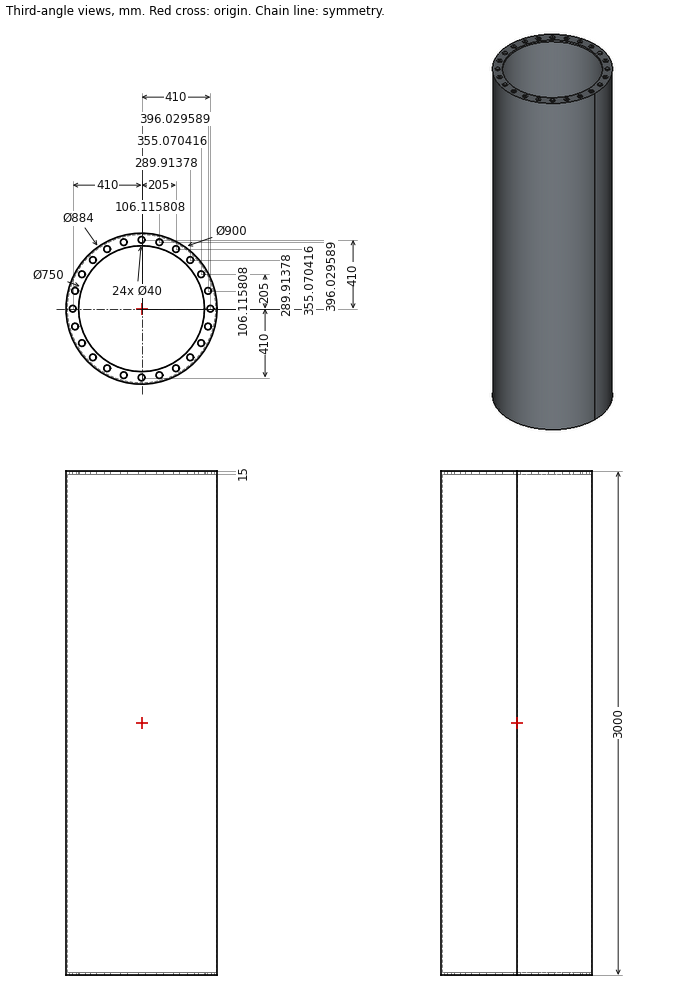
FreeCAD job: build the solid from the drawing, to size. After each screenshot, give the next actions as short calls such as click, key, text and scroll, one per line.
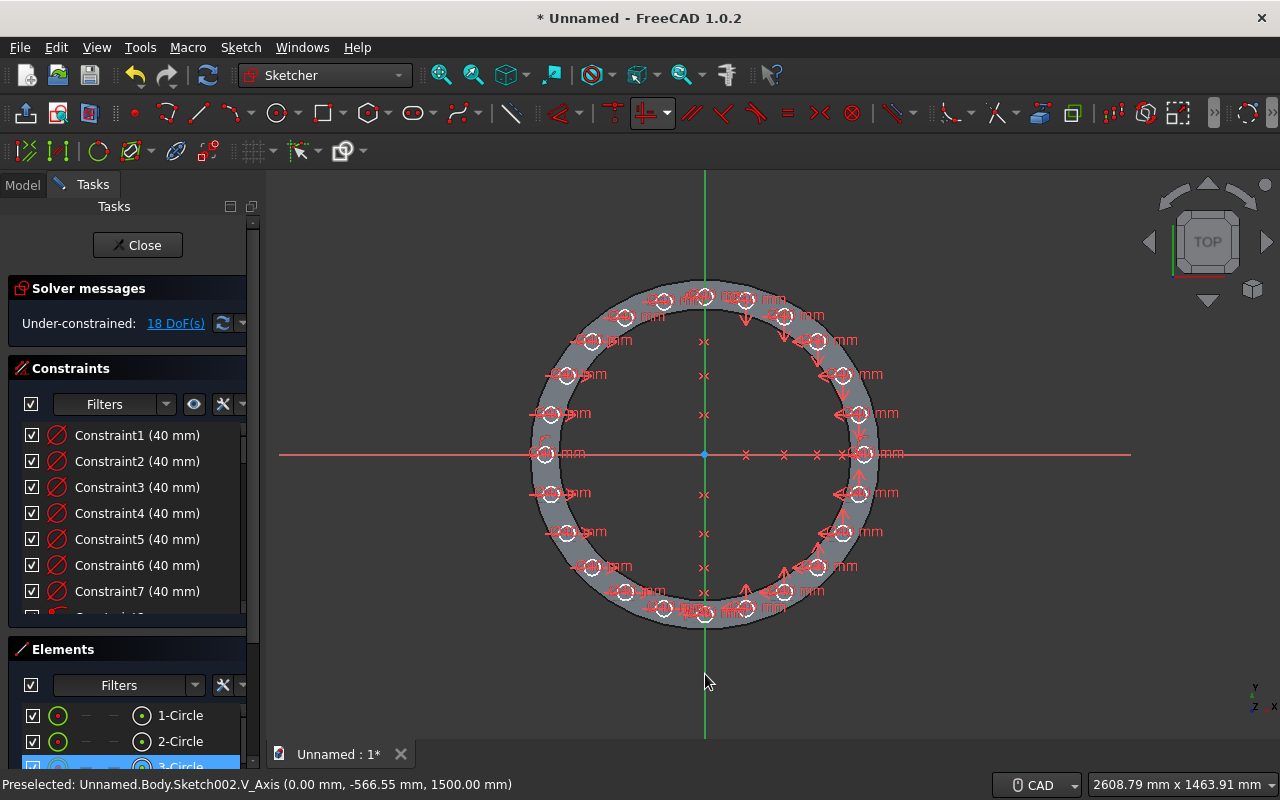
click(820, 114)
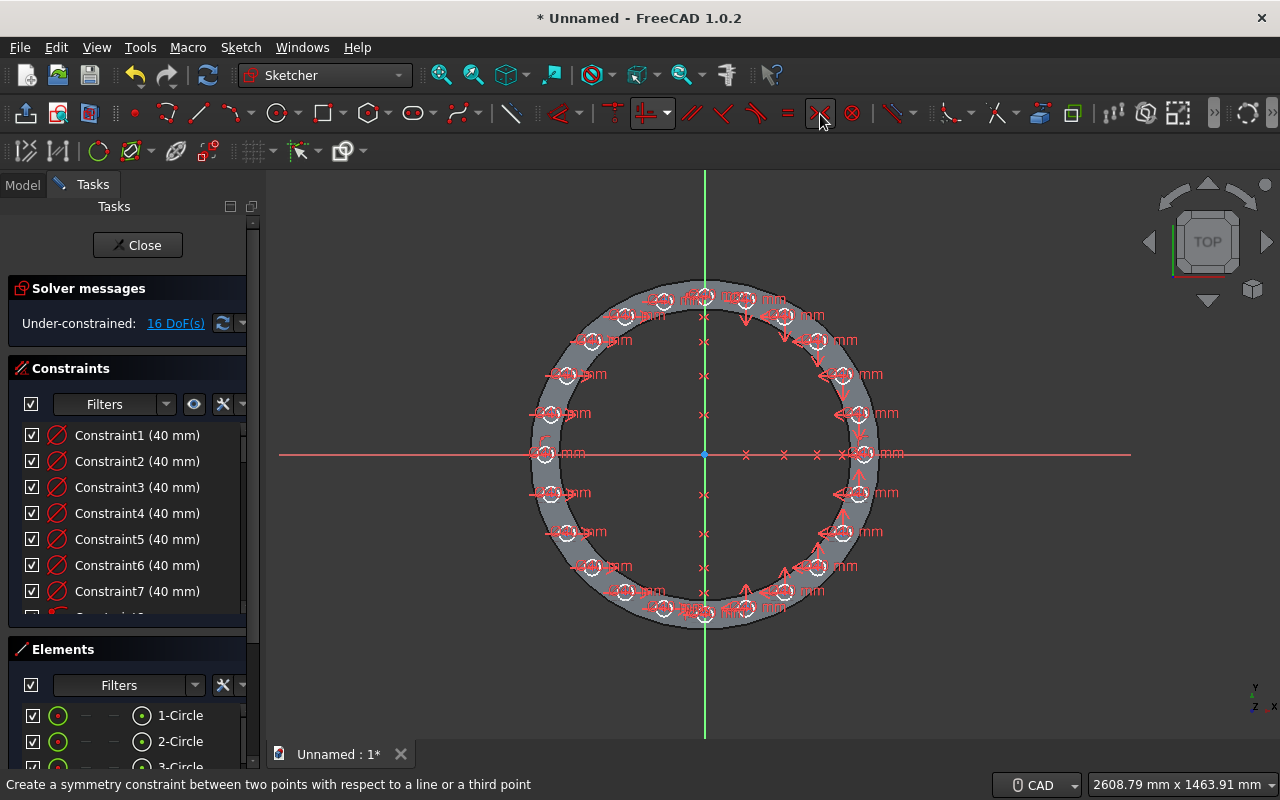
click(746, 301)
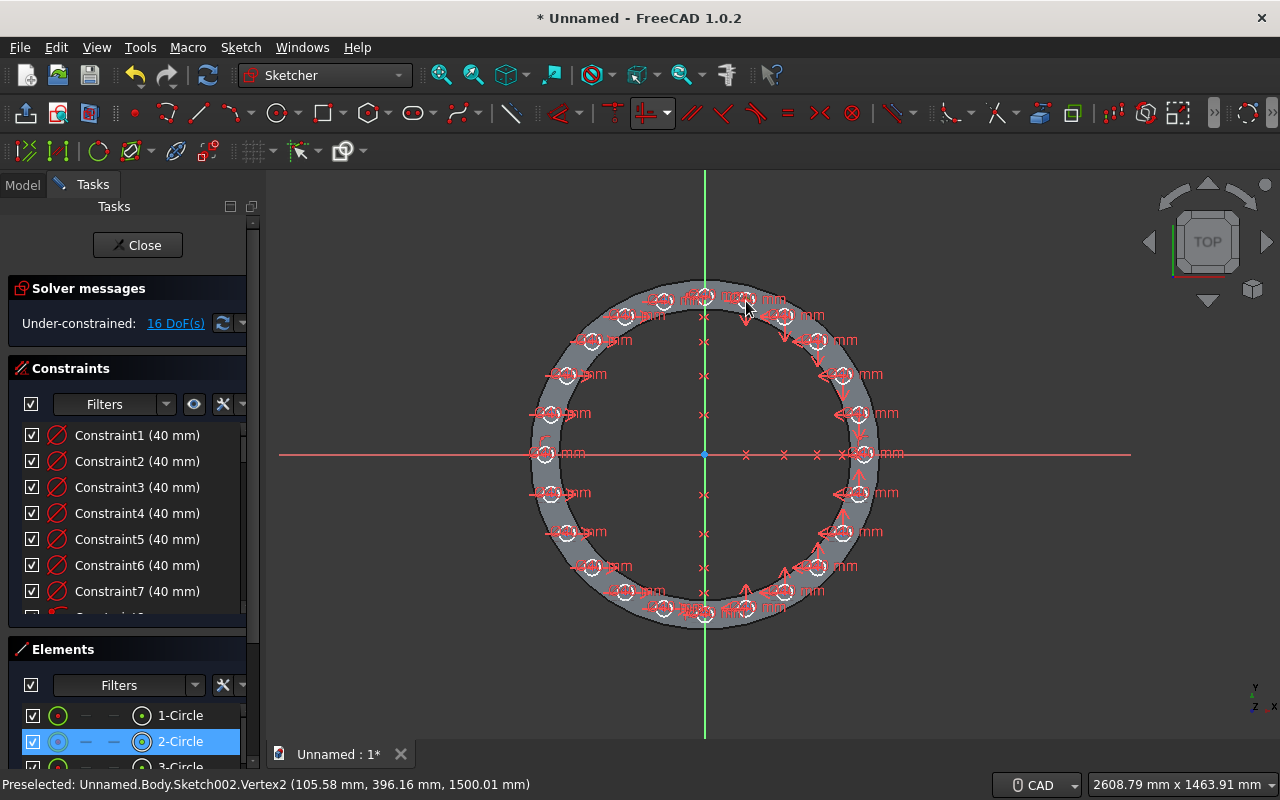
click(664, 302)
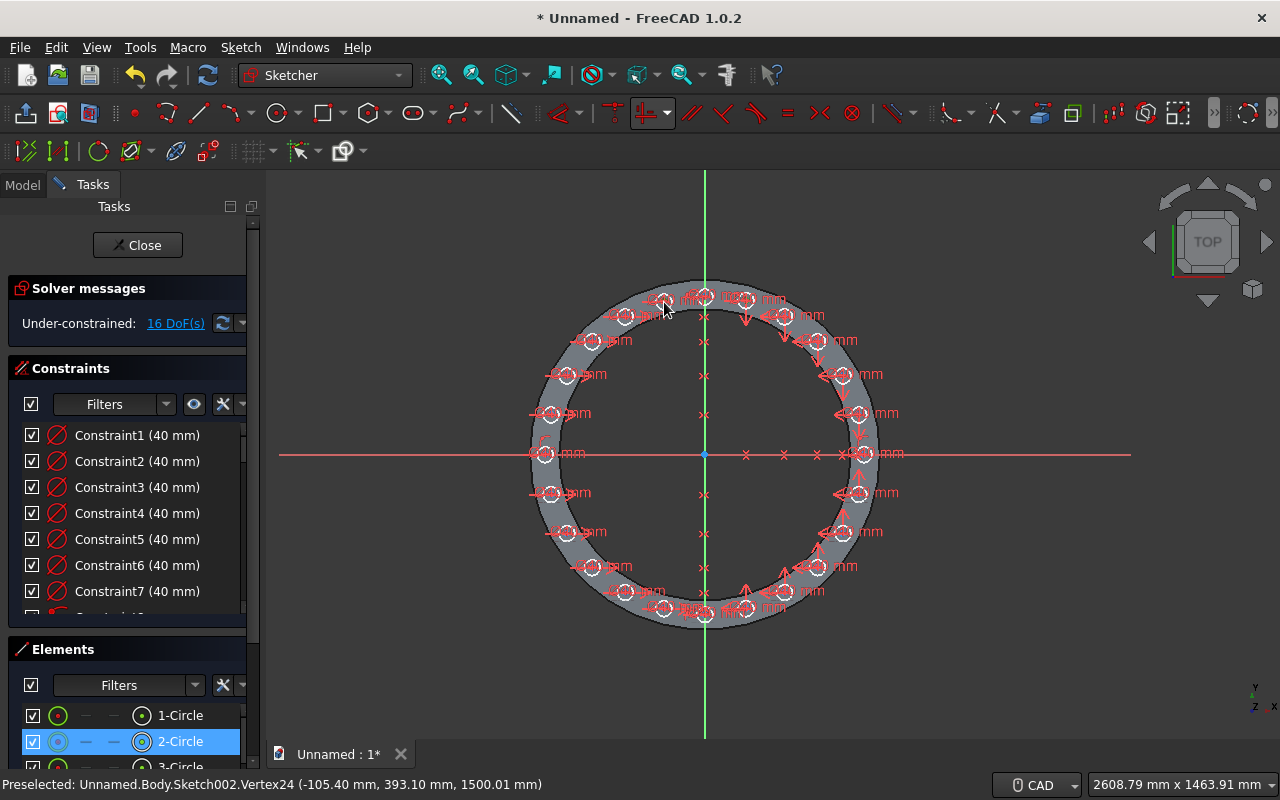
click(705, 674)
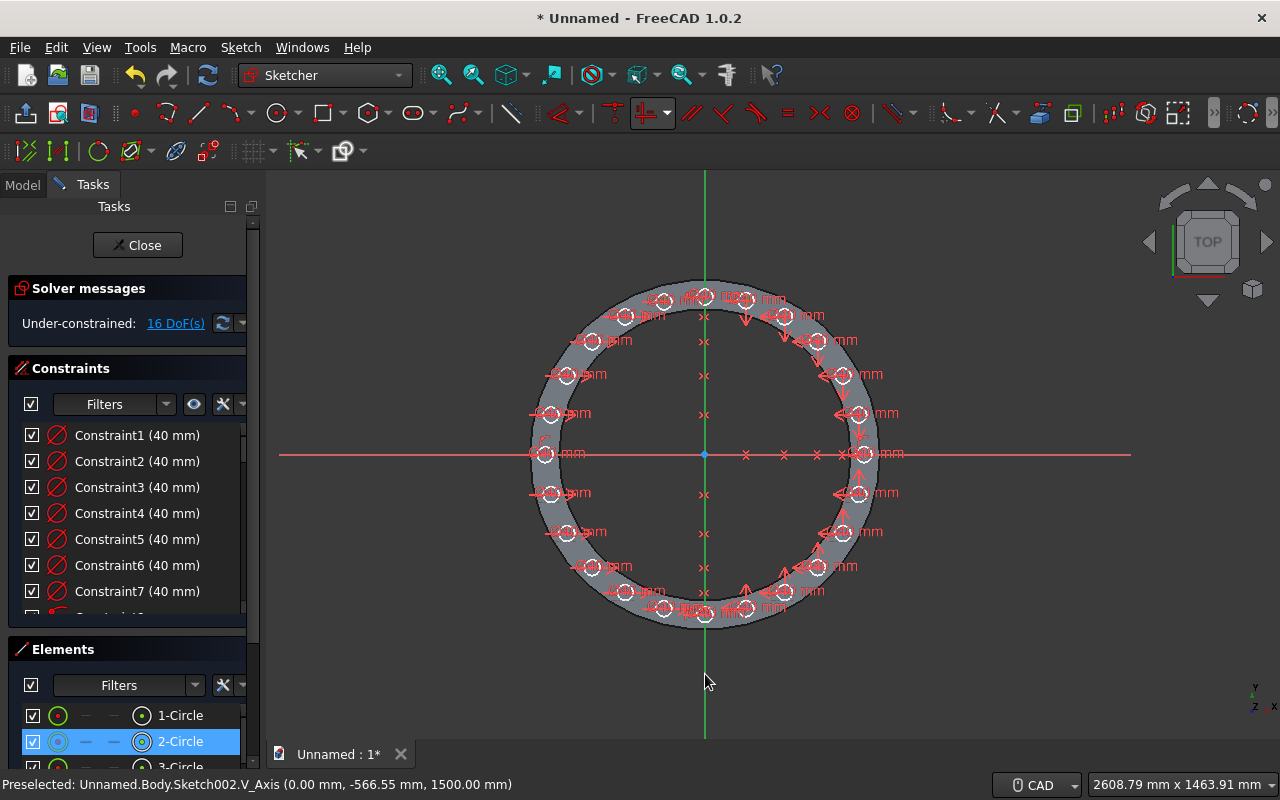
click(820, 114)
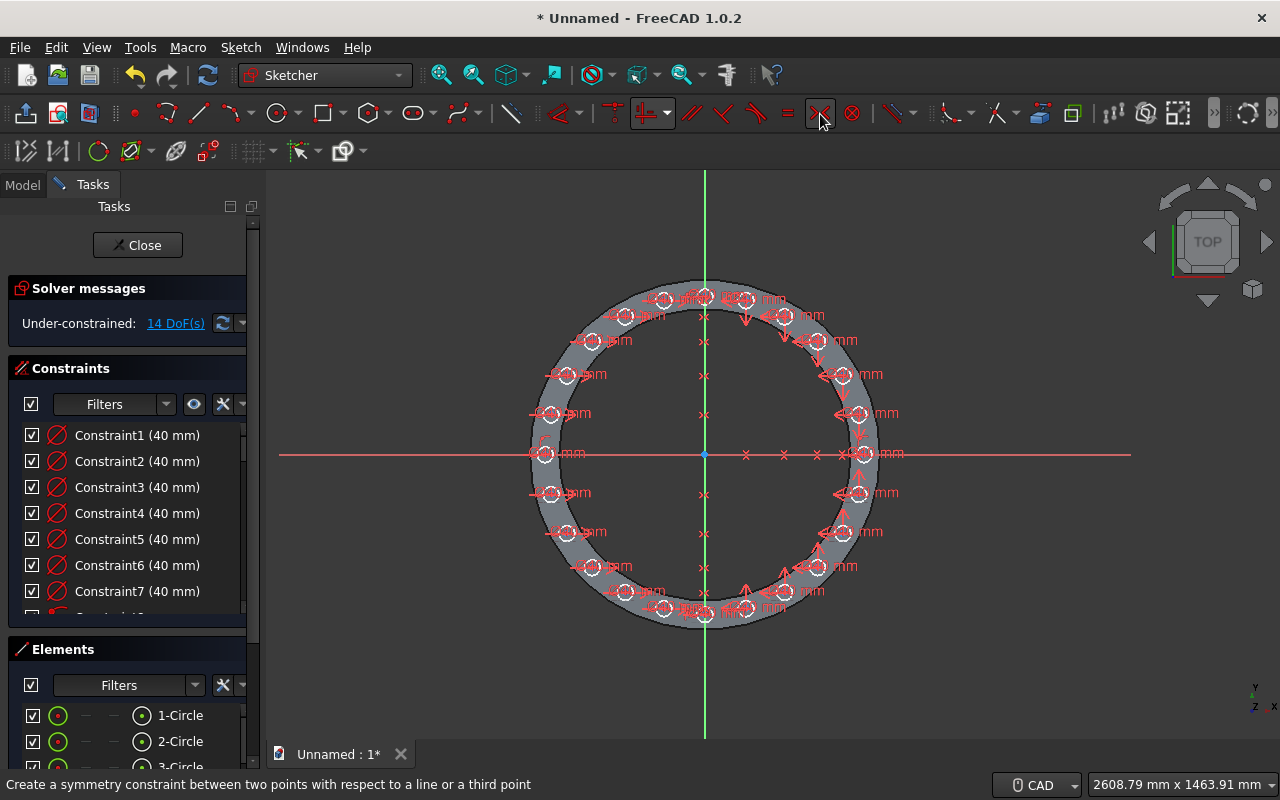
click(558, 114)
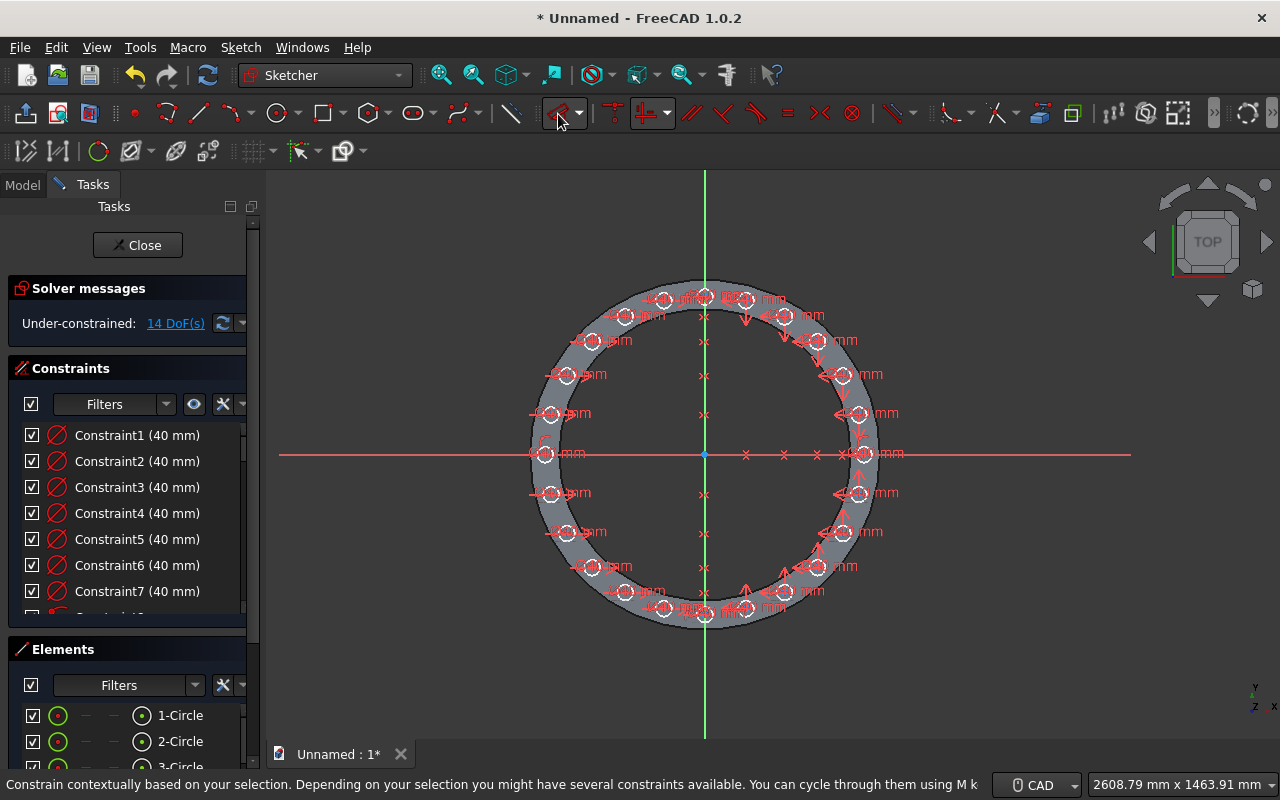
click(705, 297)
click(739, 376)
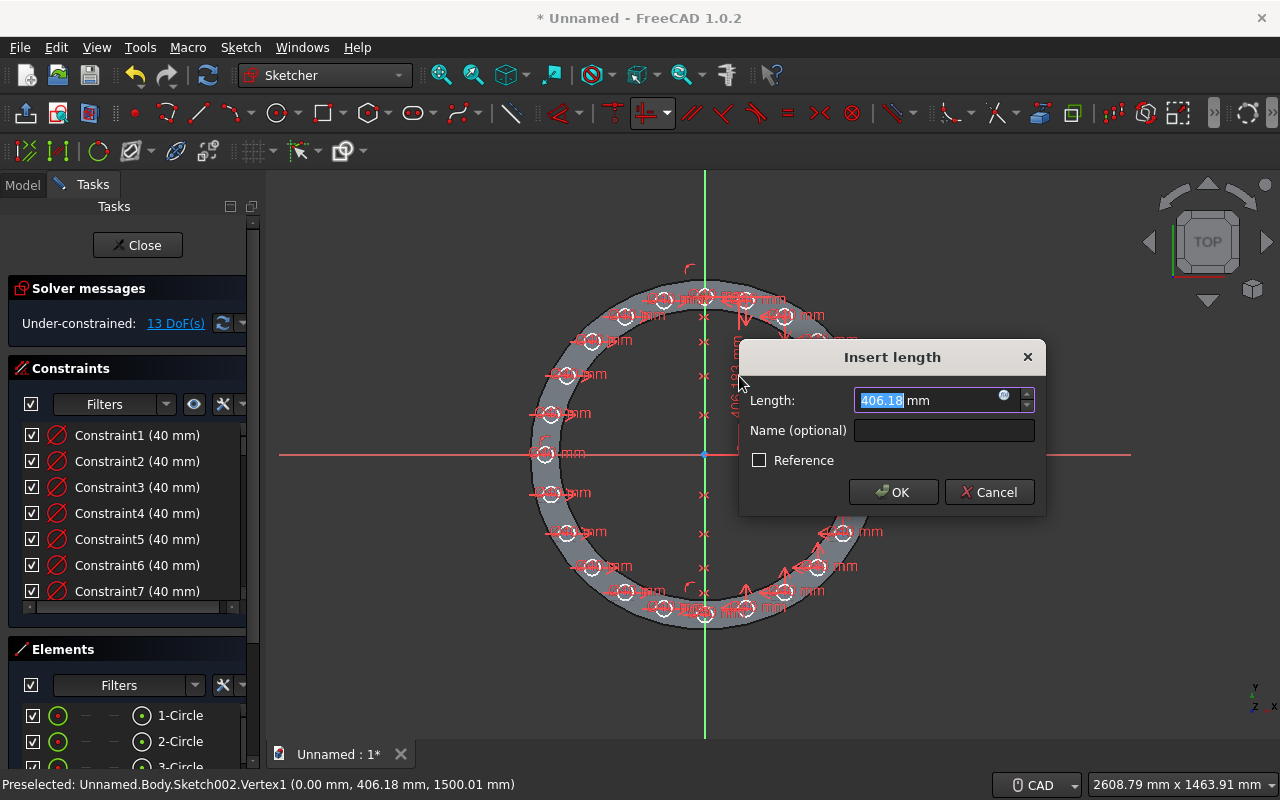
text(410)
key(Return)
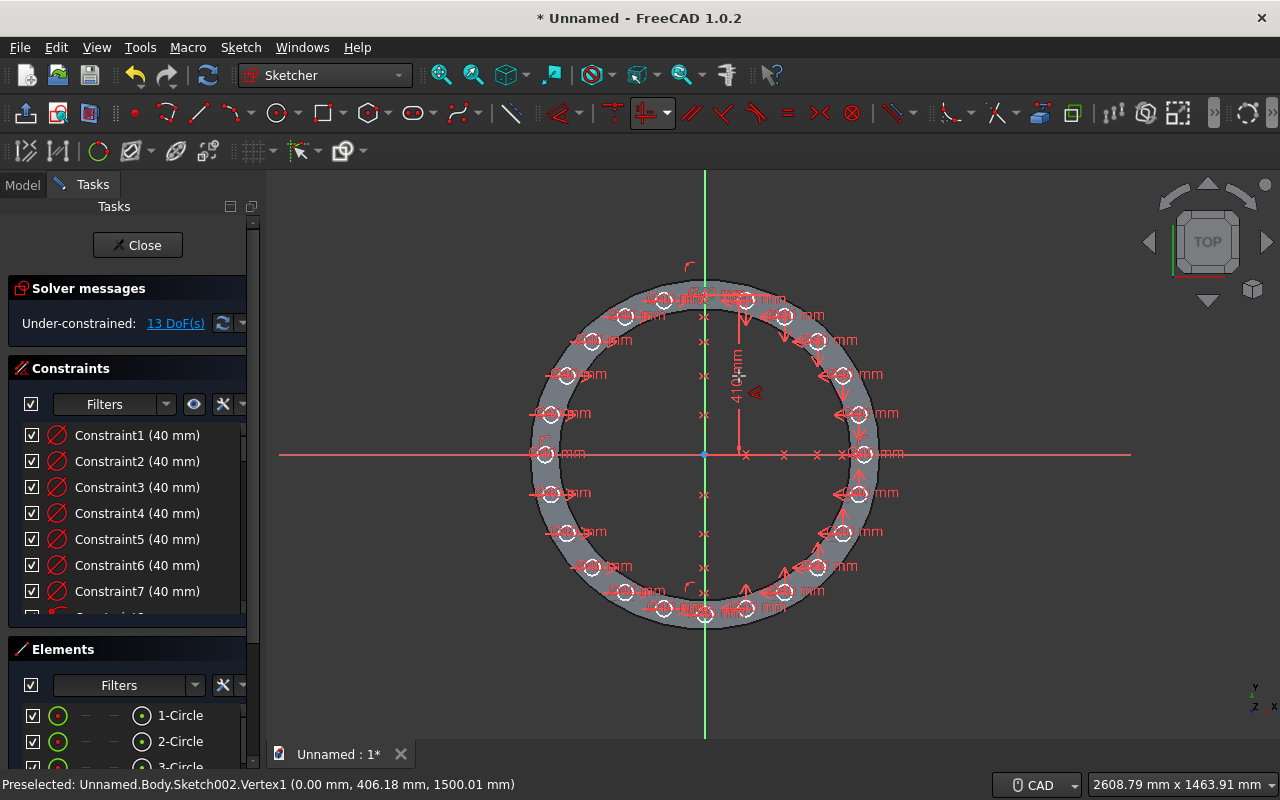
click(785, 317)
click(726, 283)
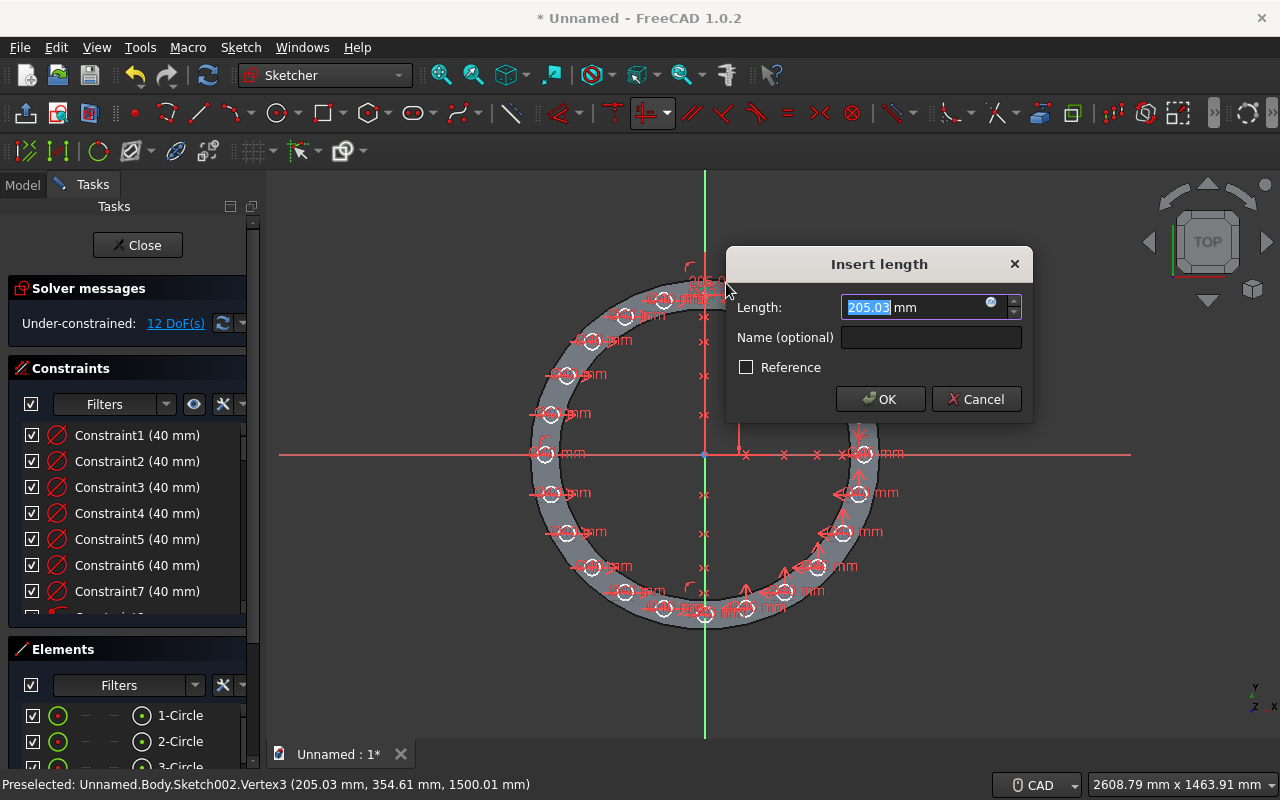
text(205)
key(Return)